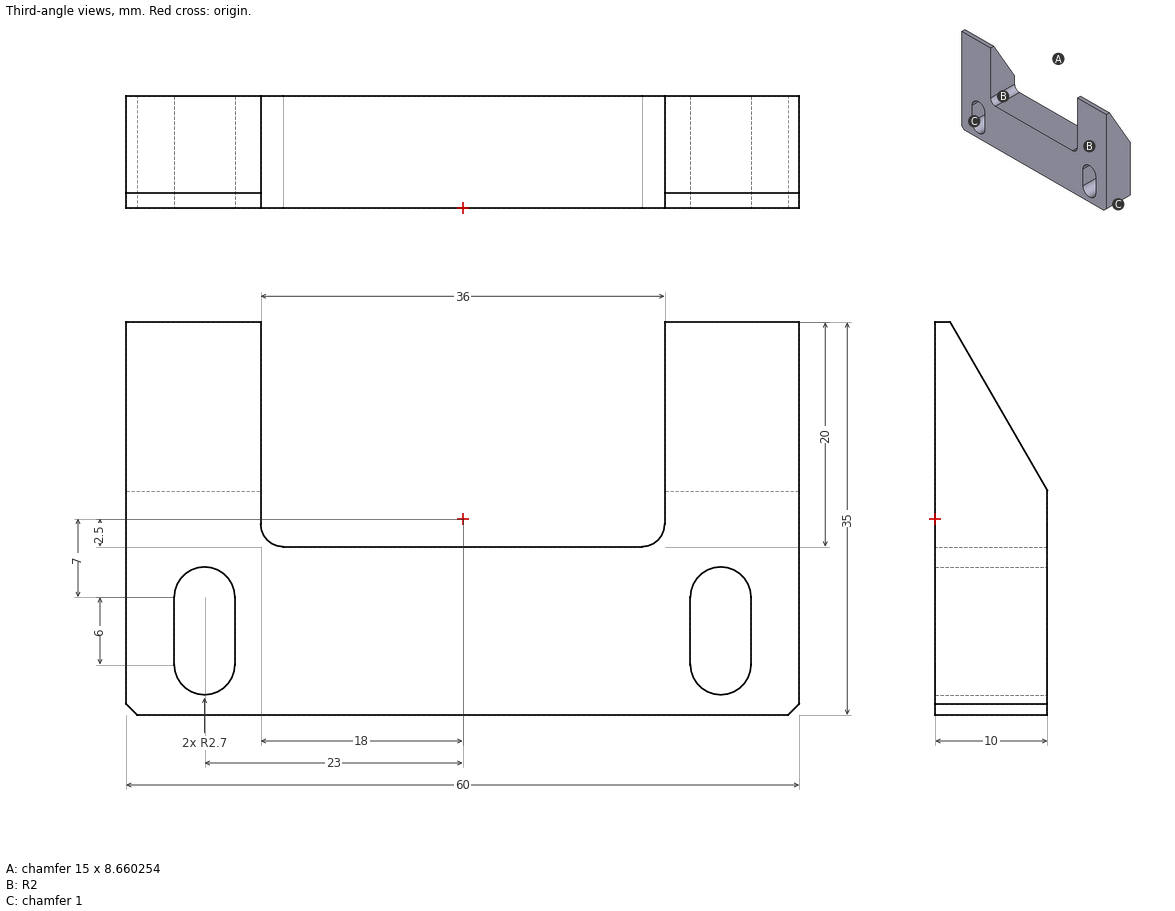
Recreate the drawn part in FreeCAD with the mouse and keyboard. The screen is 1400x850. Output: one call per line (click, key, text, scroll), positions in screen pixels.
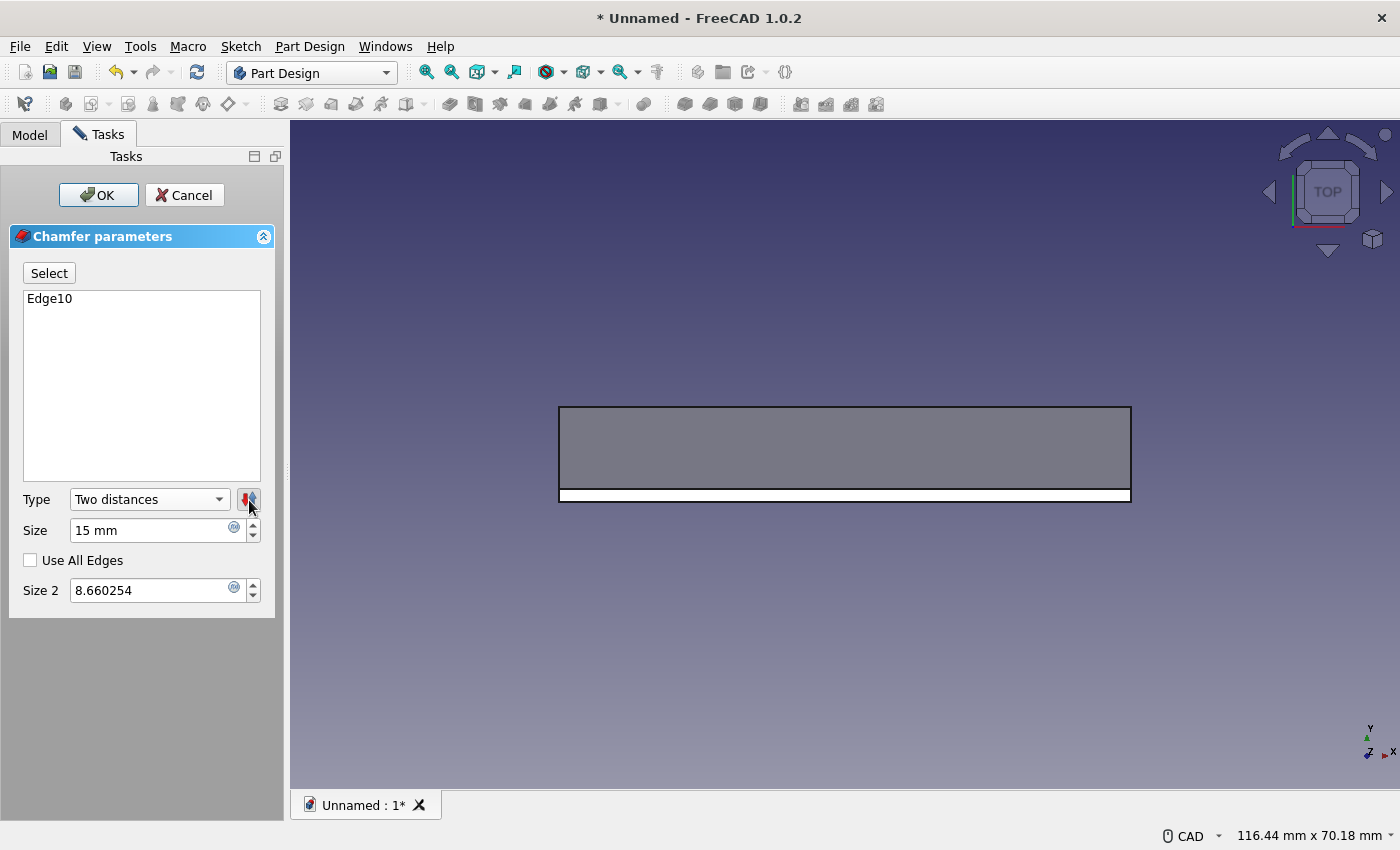
click(99, 195)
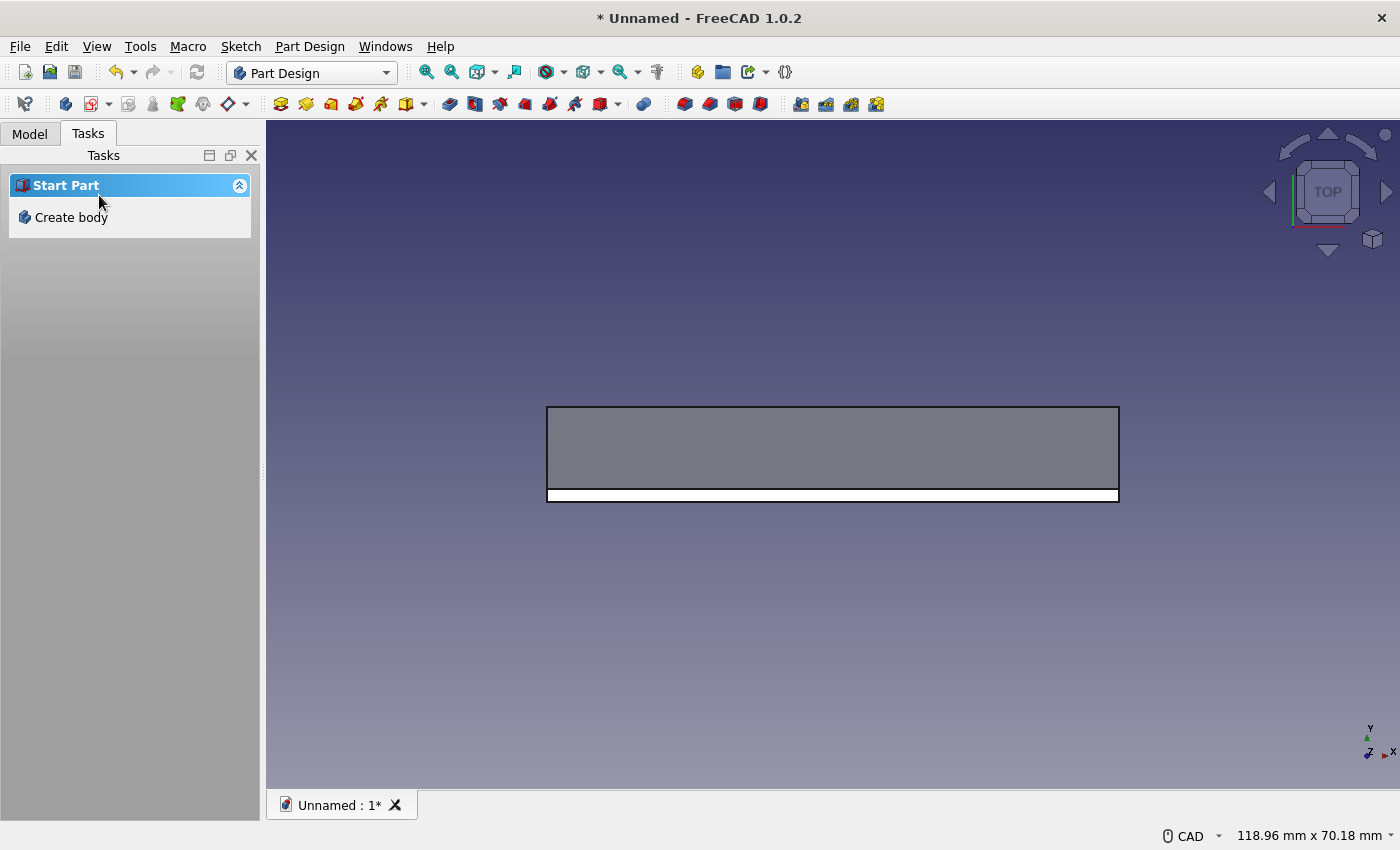
key(4)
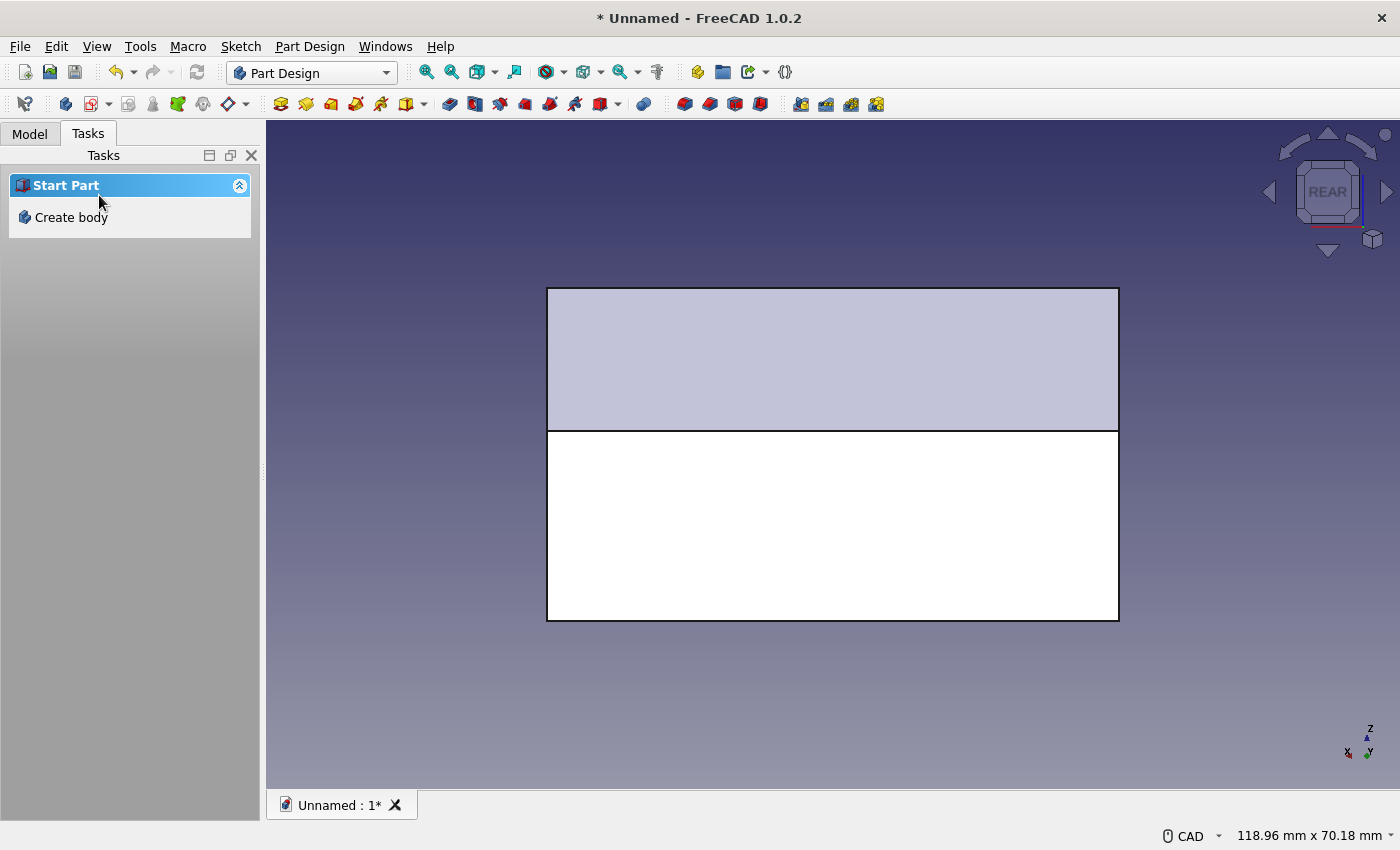
click(670, 525)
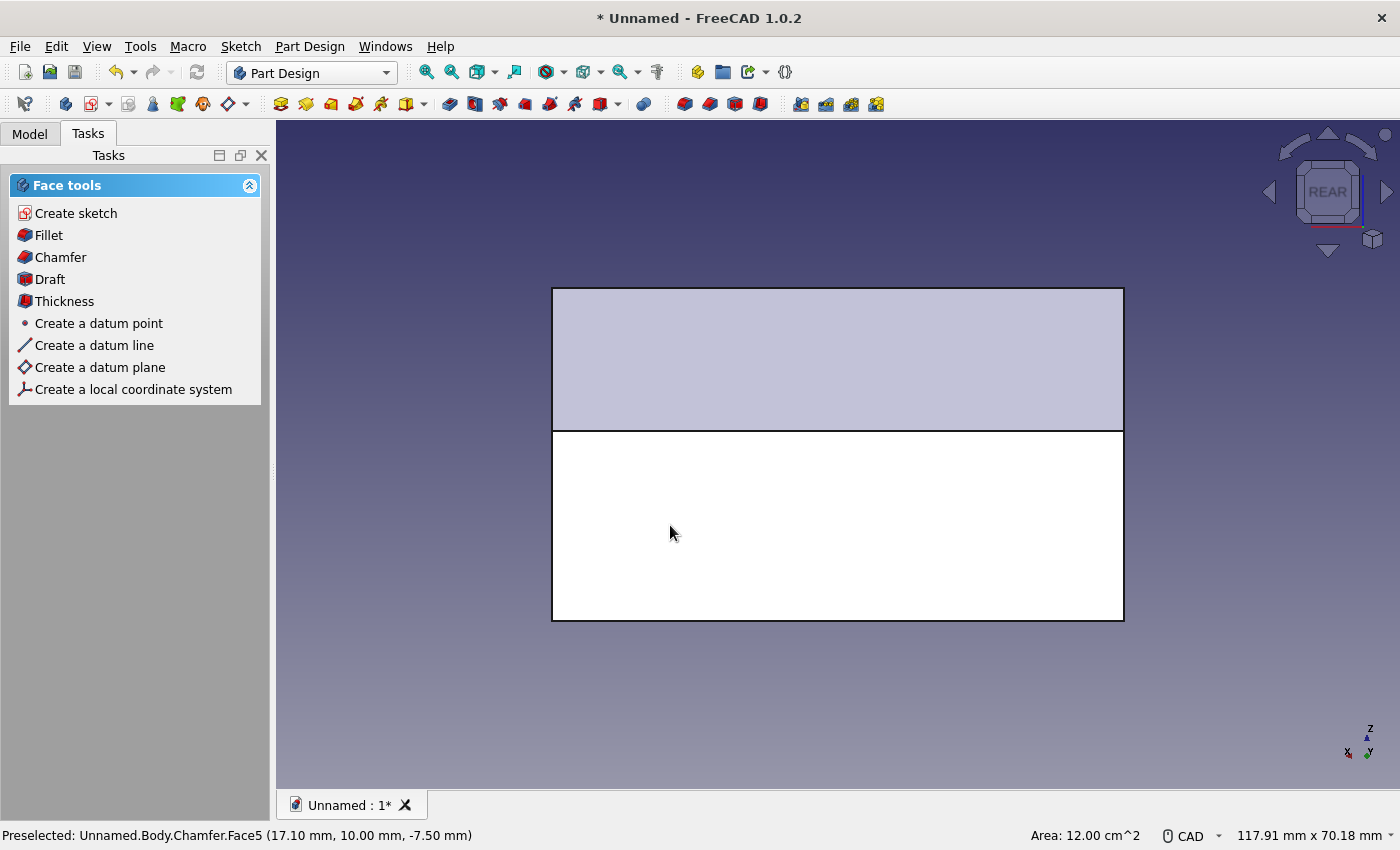
click(90, 104)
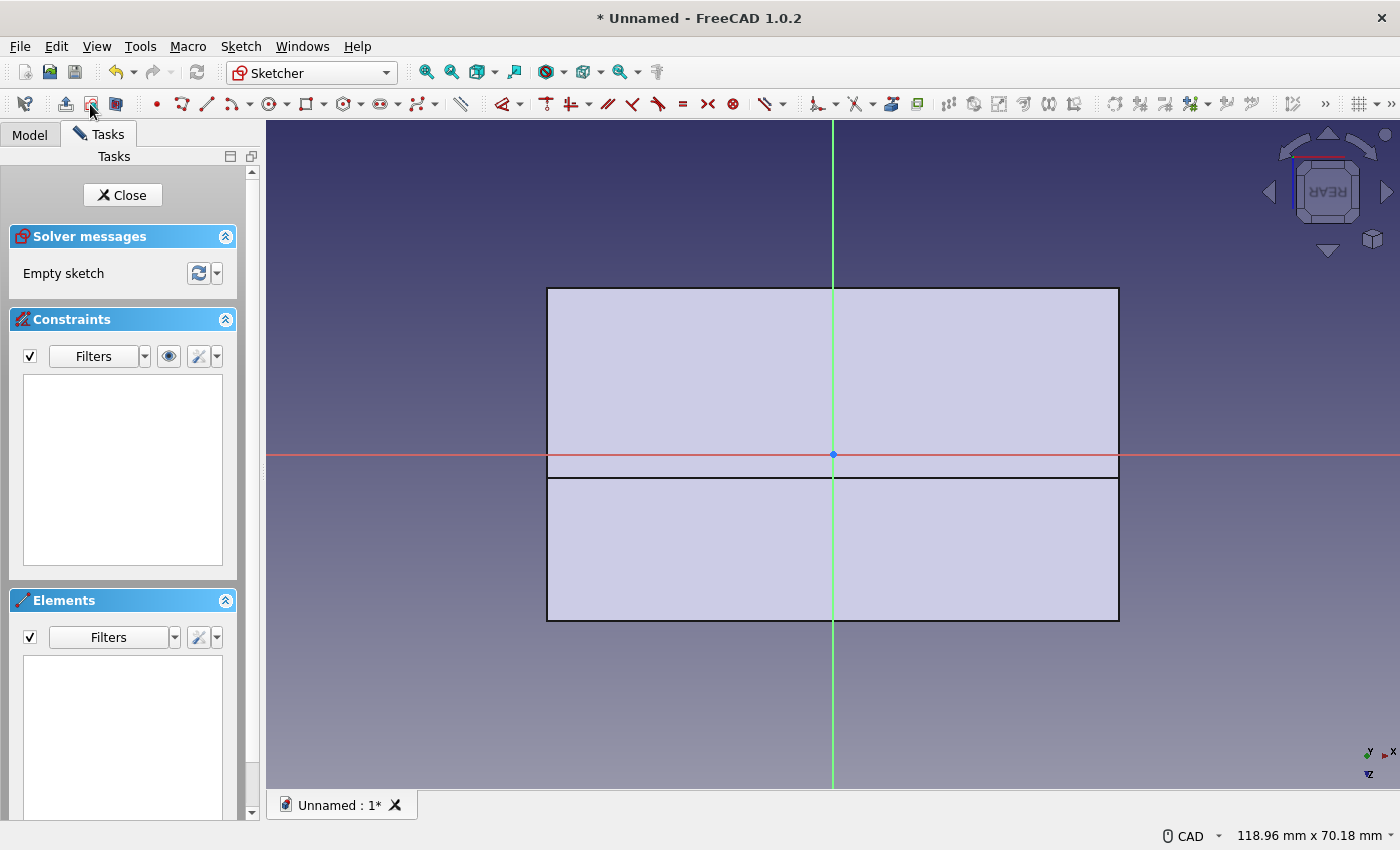
scroll(916, 613, up, 3)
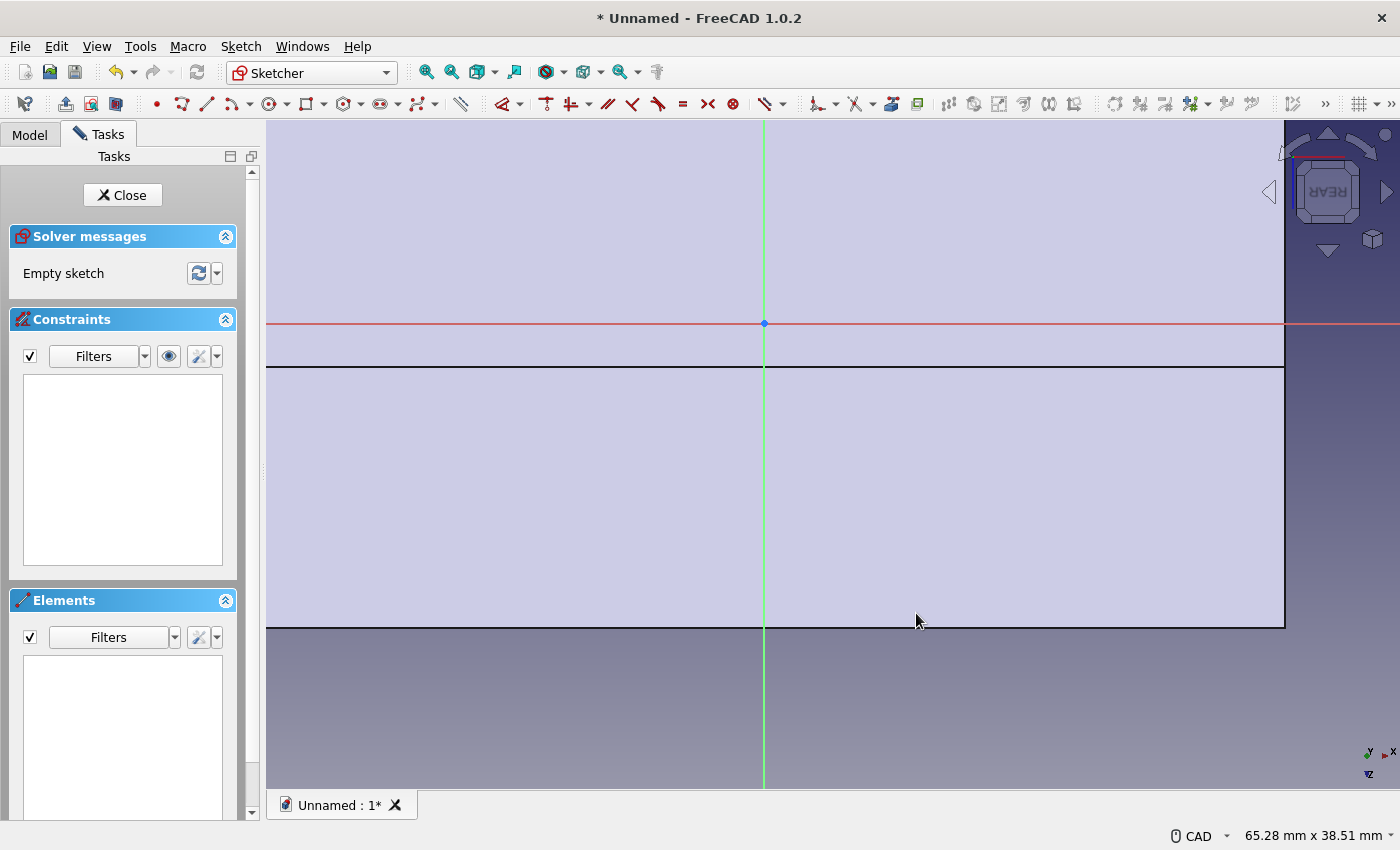
click(306, 104)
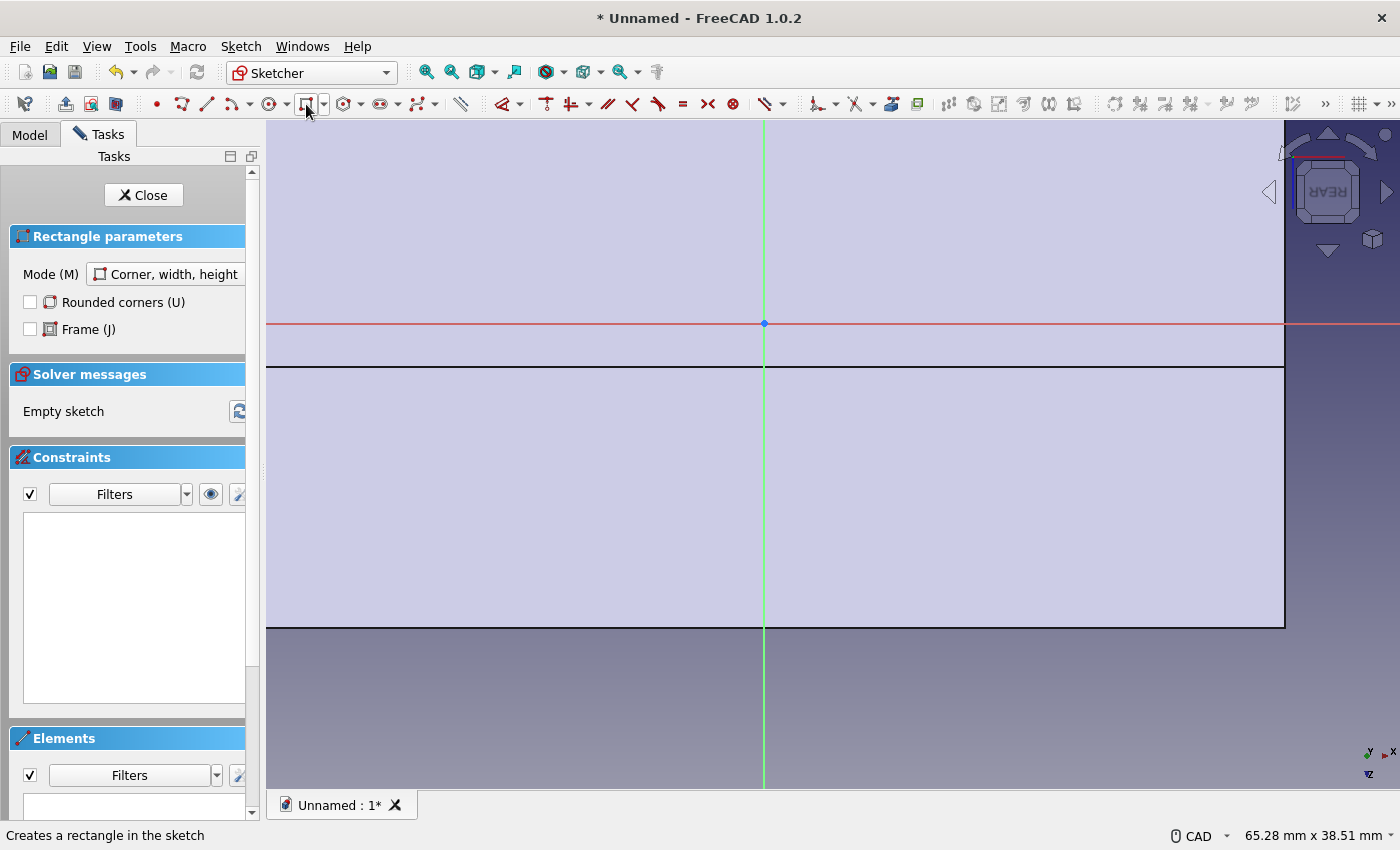
click(452, 280)
move(1077, 628)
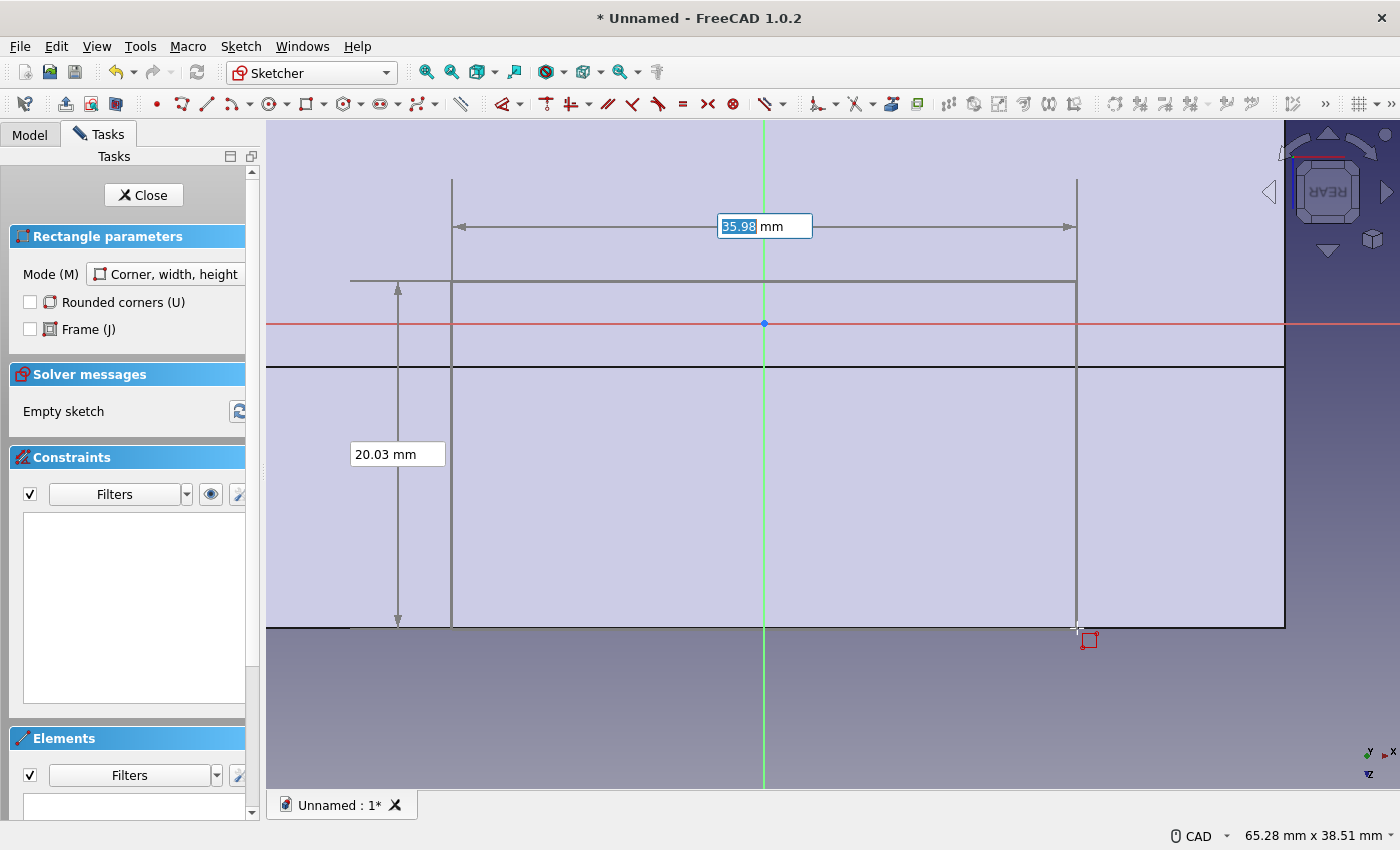
text(36)
key(Tab)
text(20)
key(Return)
key(Escape)